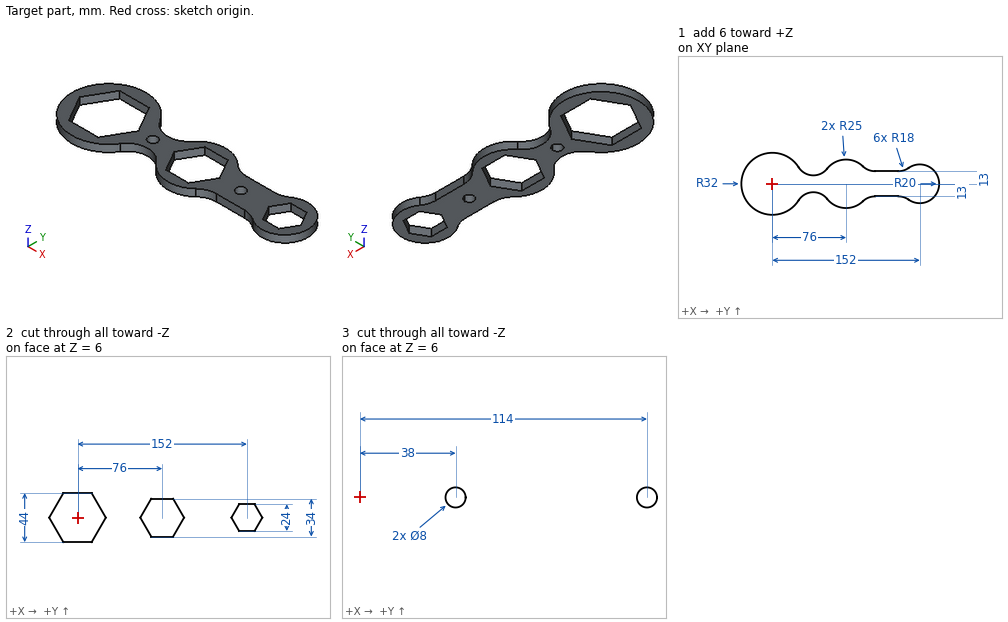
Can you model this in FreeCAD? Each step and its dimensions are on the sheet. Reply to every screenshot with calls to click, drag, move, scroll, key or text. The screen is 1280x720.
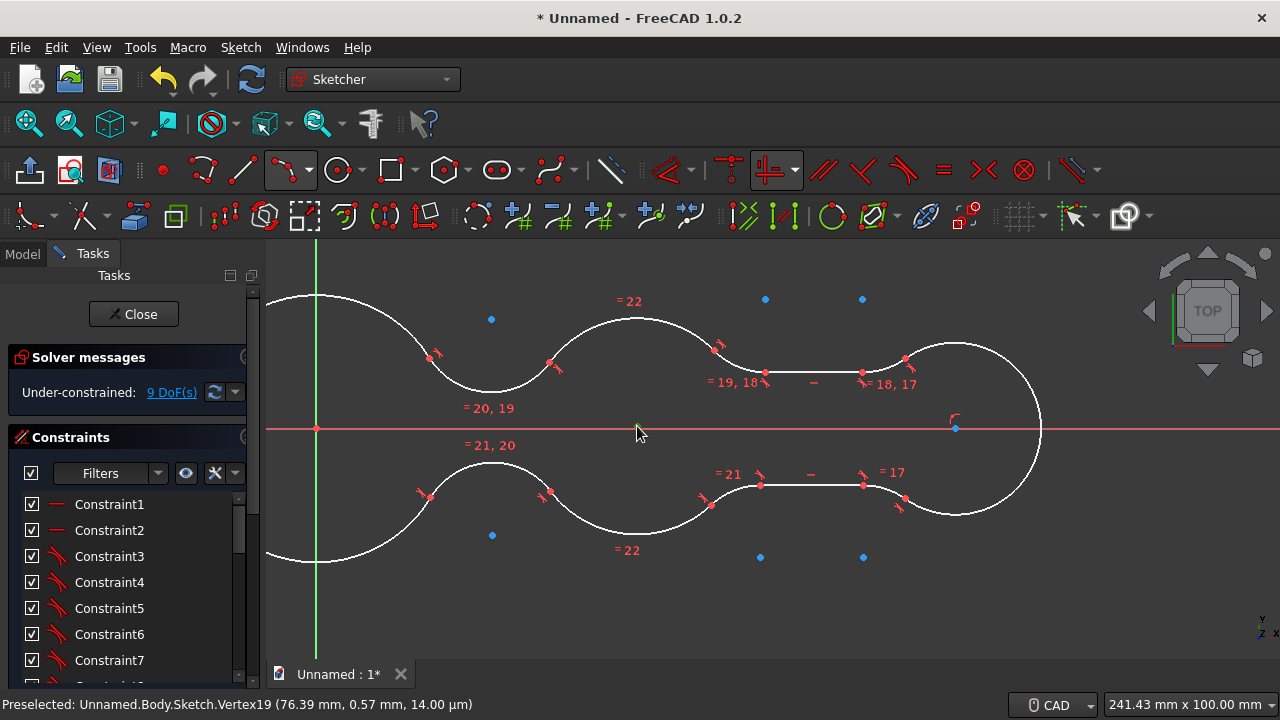
click(353, 429)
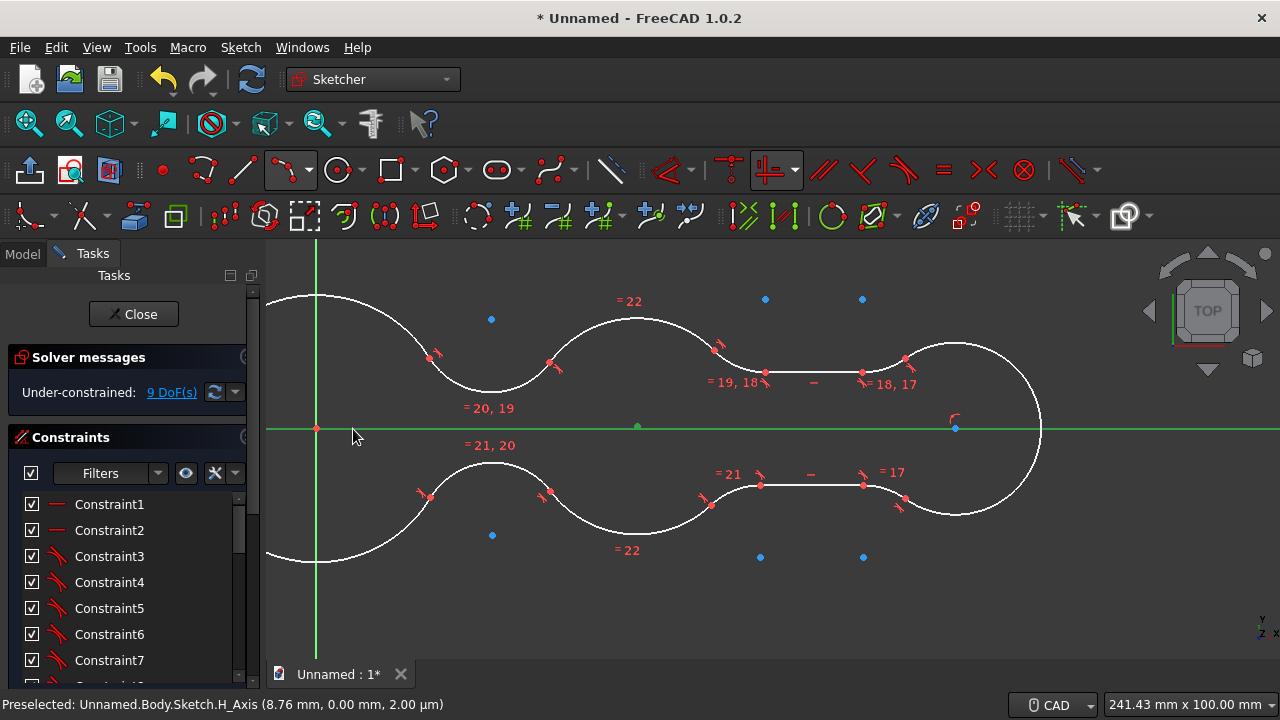
click(730, 170)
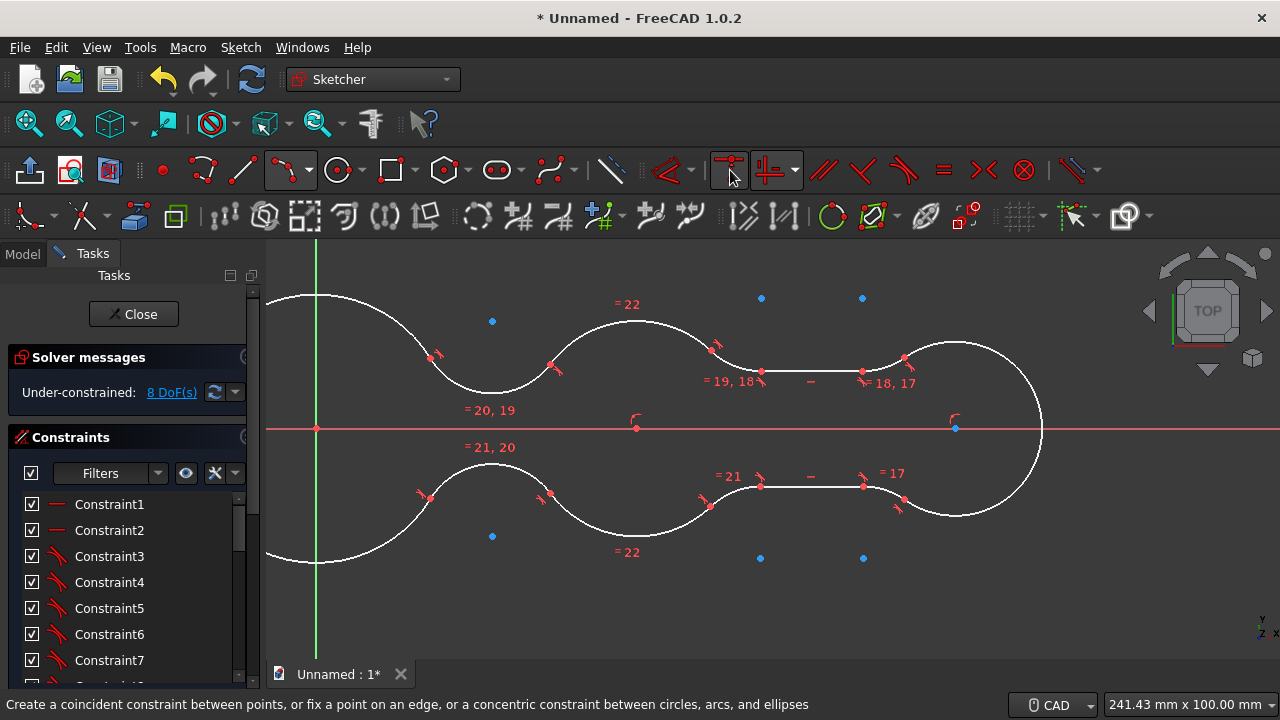
click(893, 493)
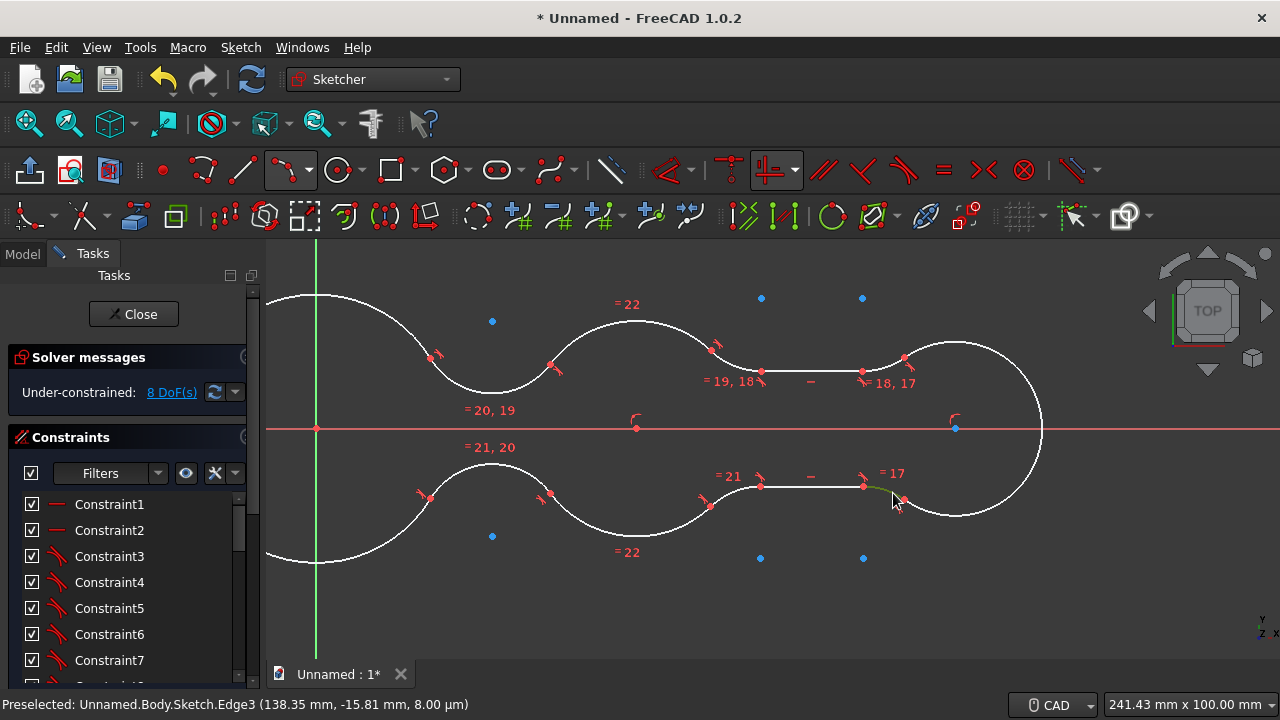
click(694, 170)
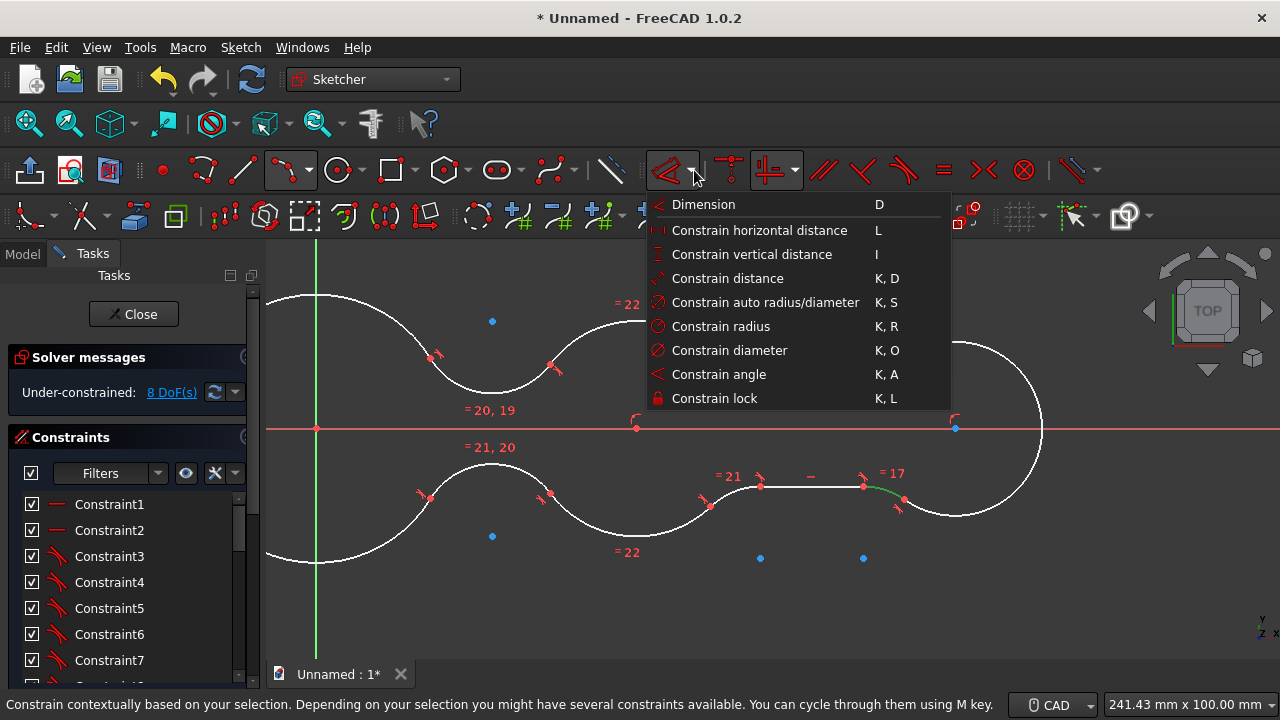
click(799, 326)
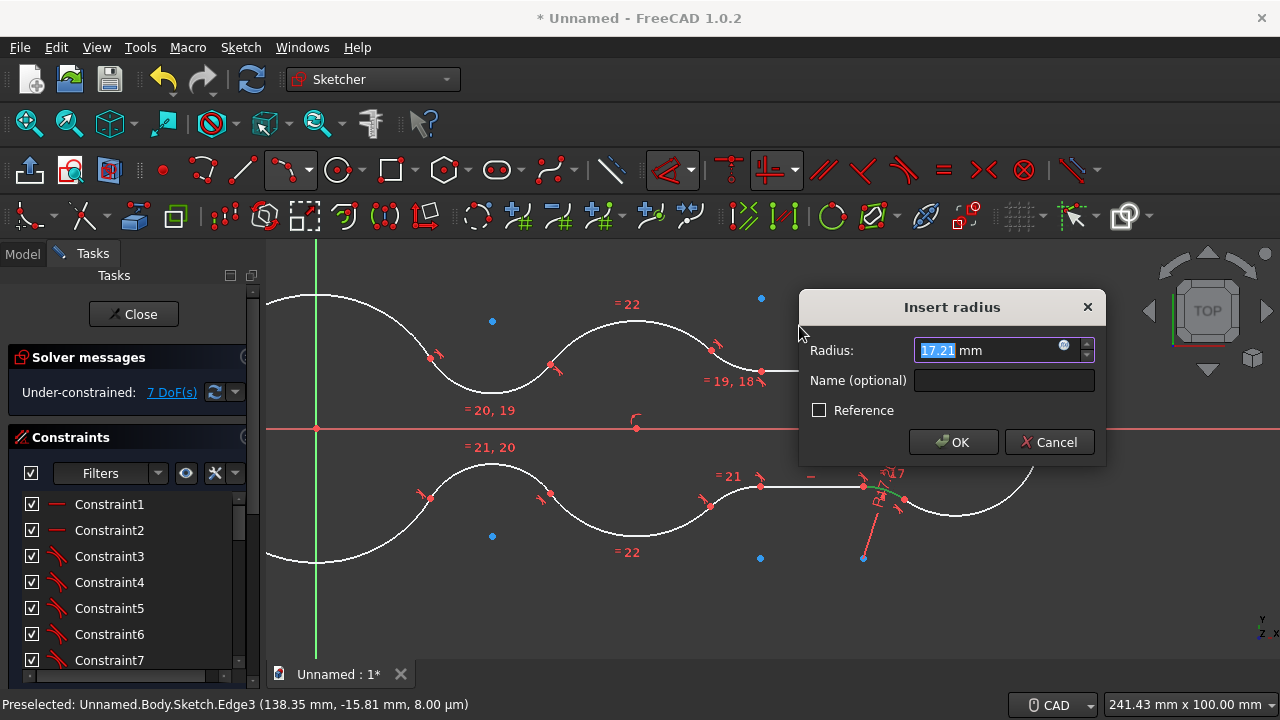
text(18)
key(Return)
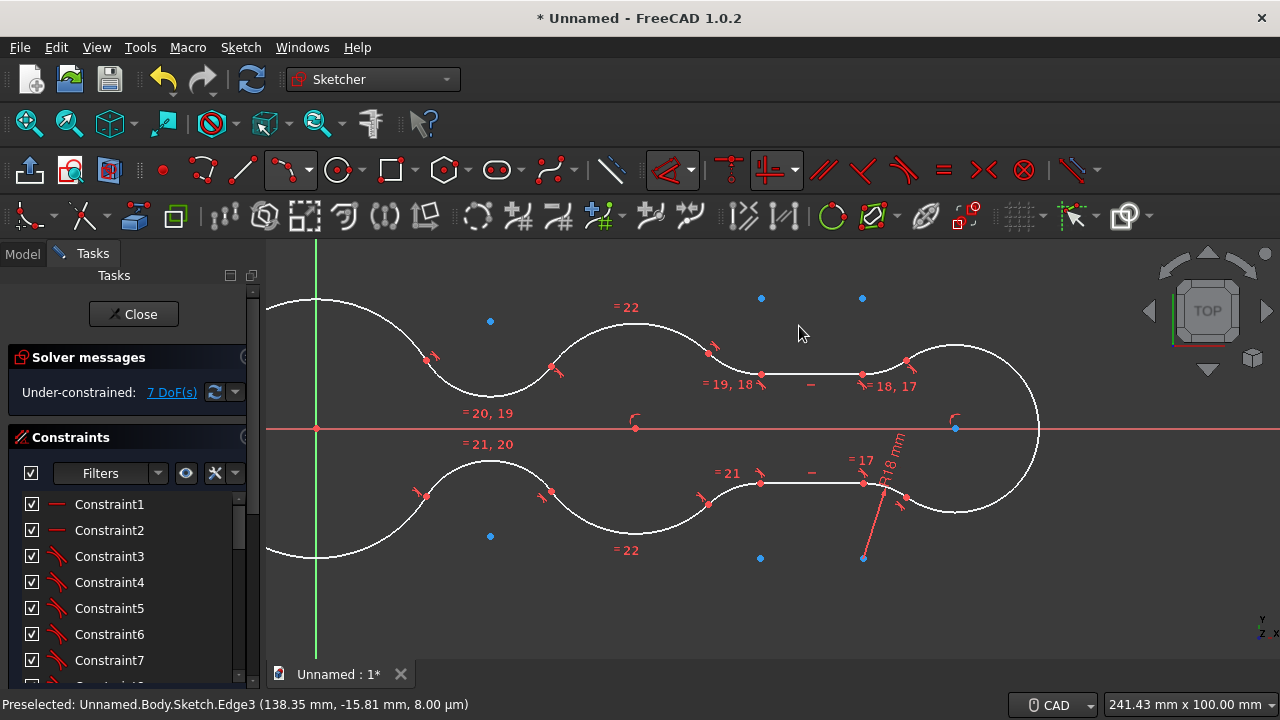
click(1009, 493)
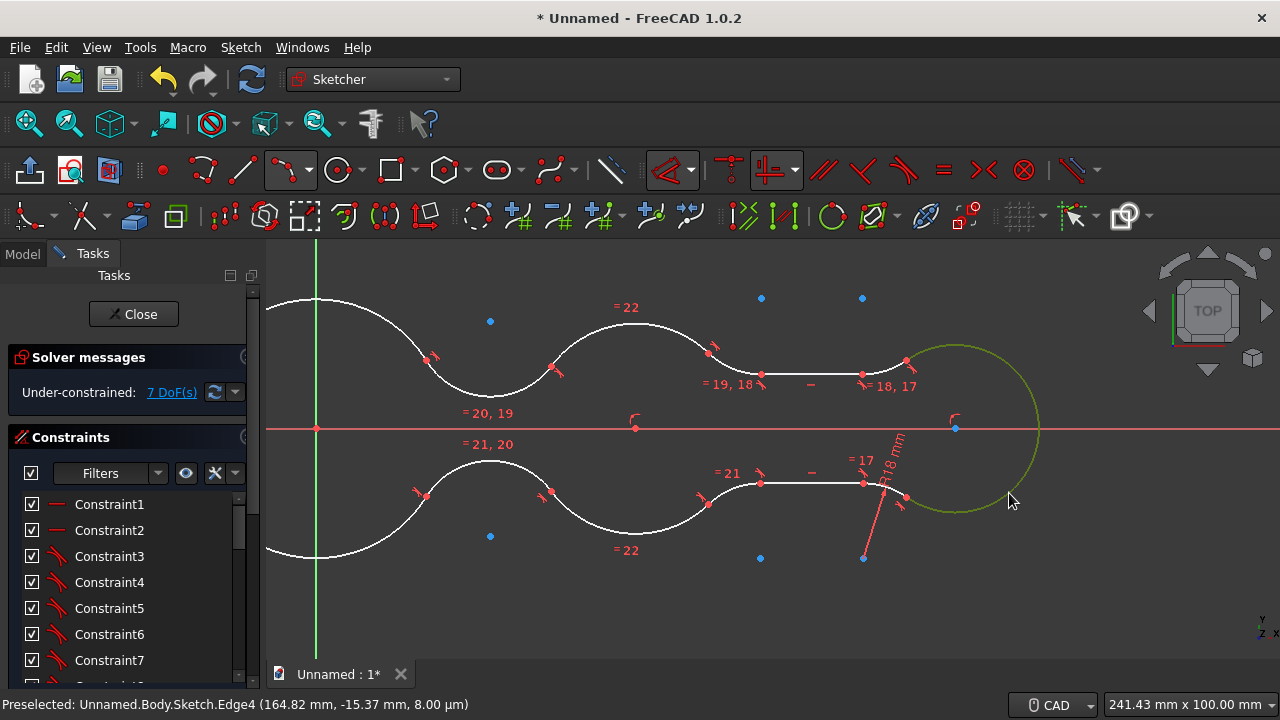
key(k)
key(r)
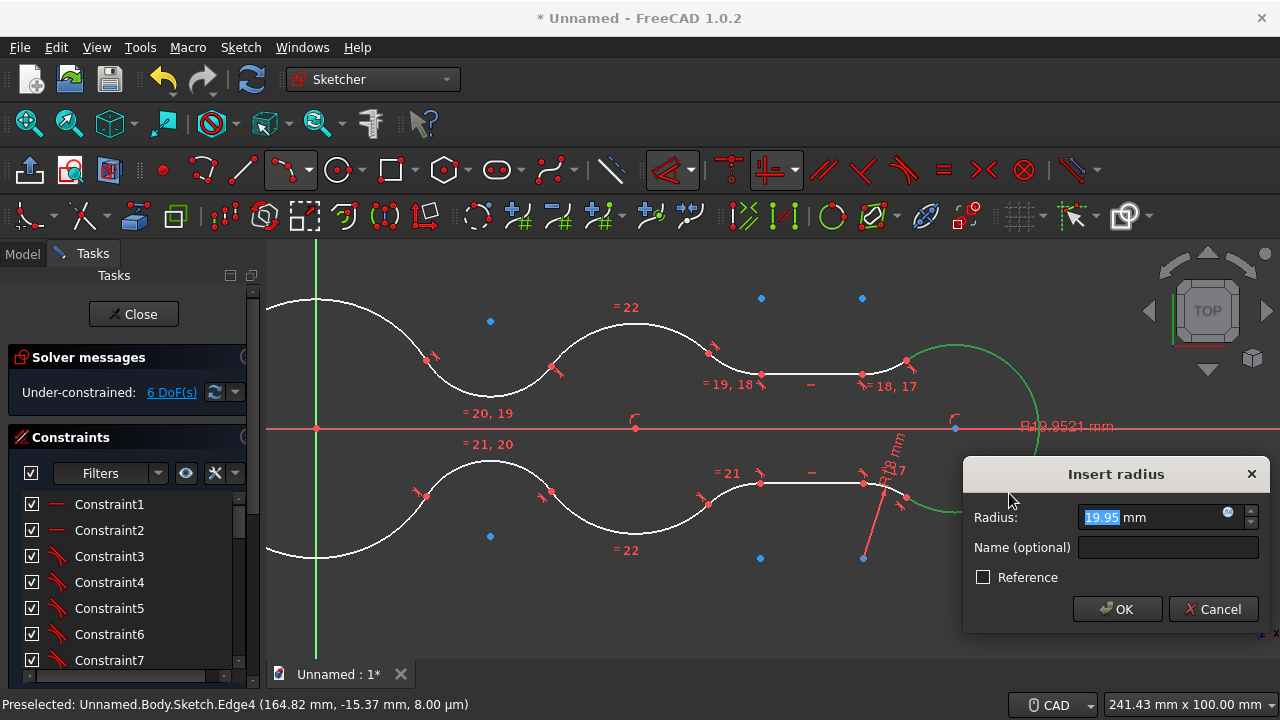
text(20)
key(Return)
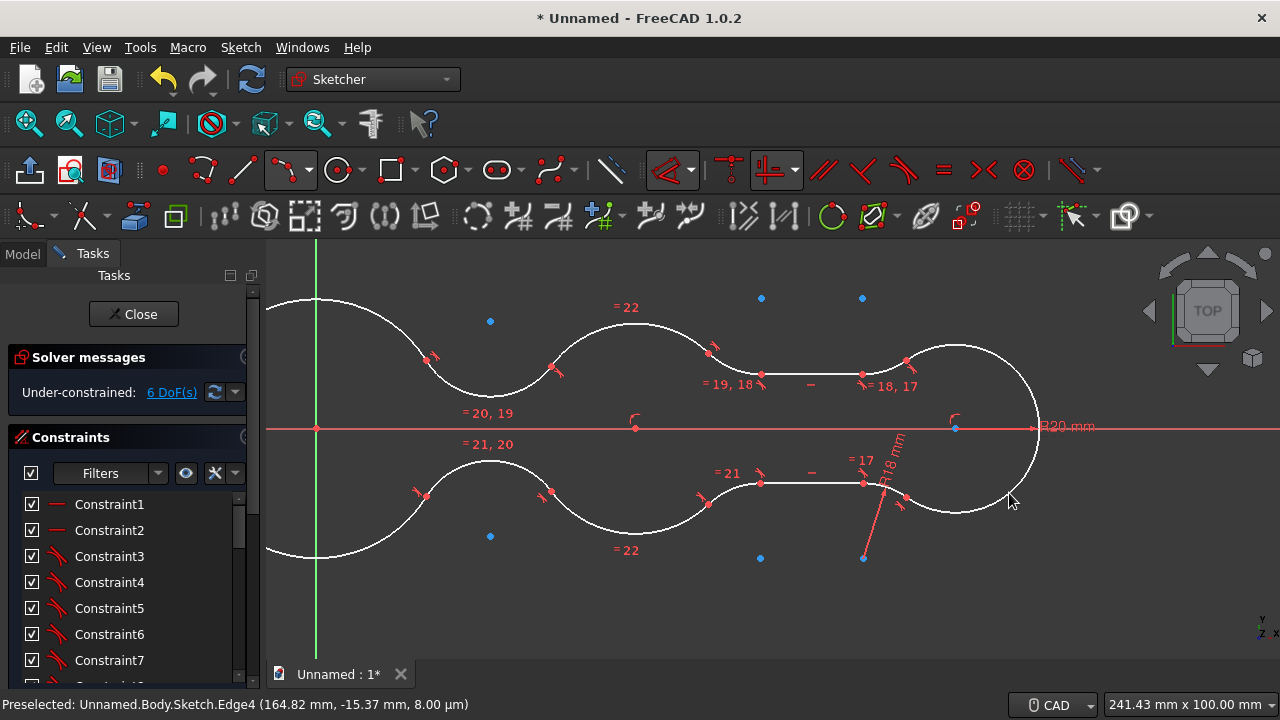
click(662, 327)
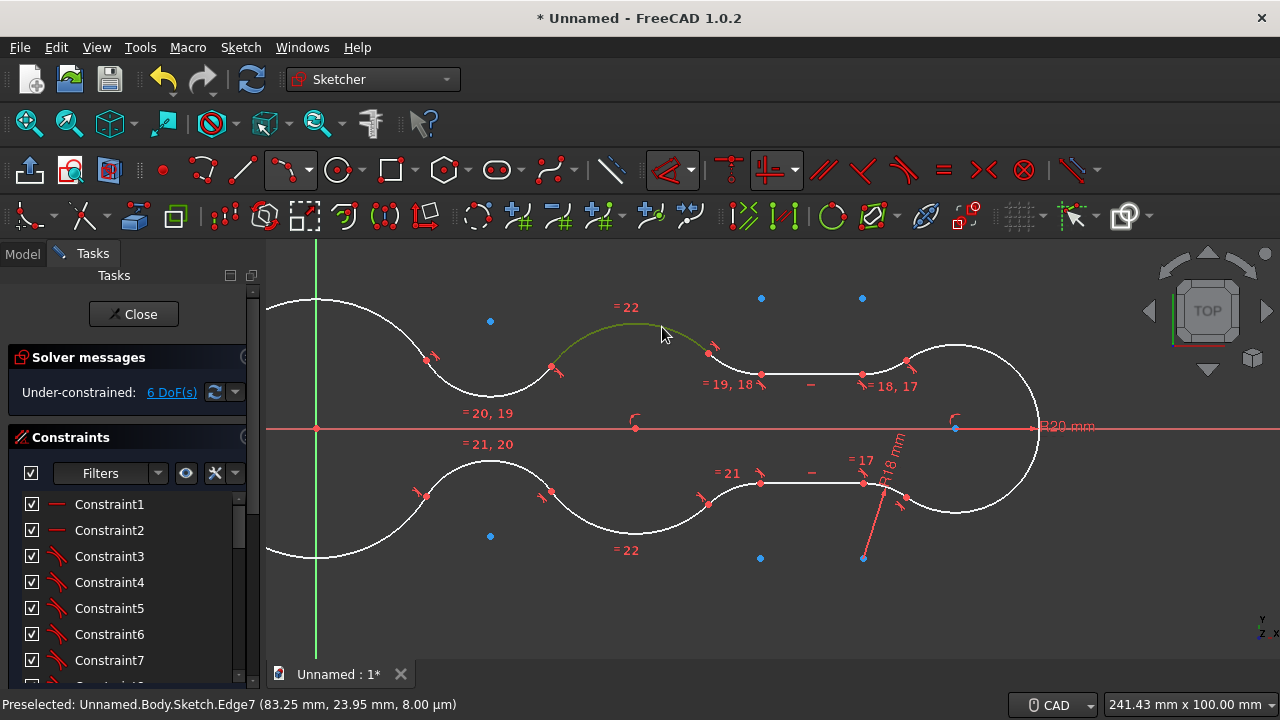
click(694, 170)